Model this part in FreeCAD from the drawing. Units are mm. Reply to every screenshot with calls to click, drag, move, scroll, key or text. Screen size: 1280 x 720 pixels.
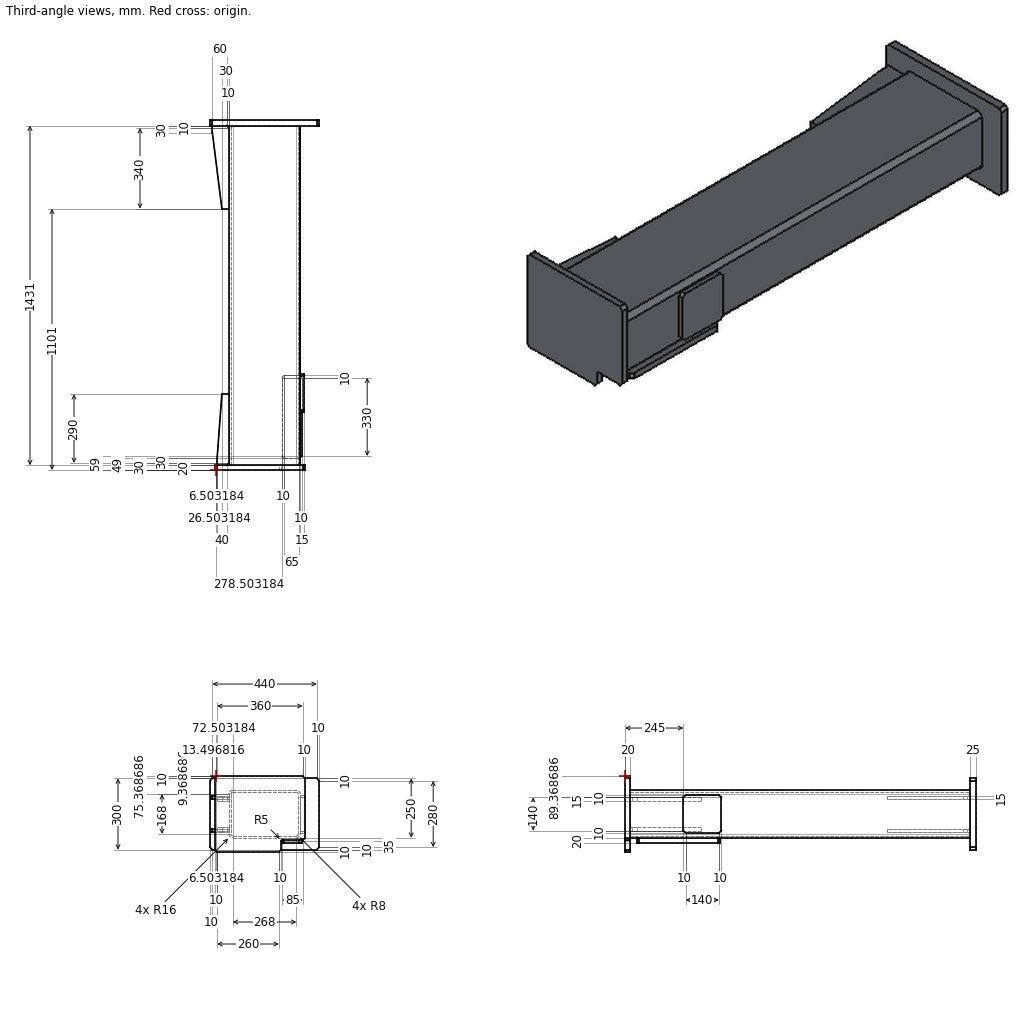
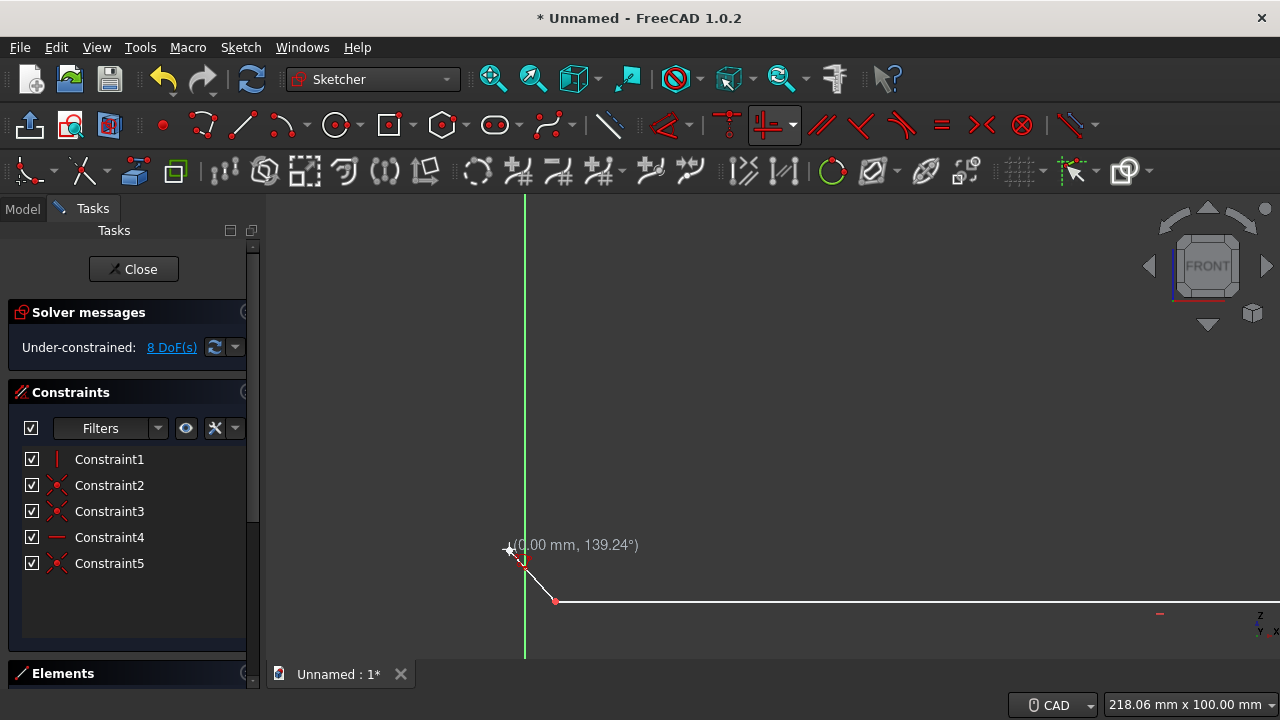
scroll(530, 572, down, 8)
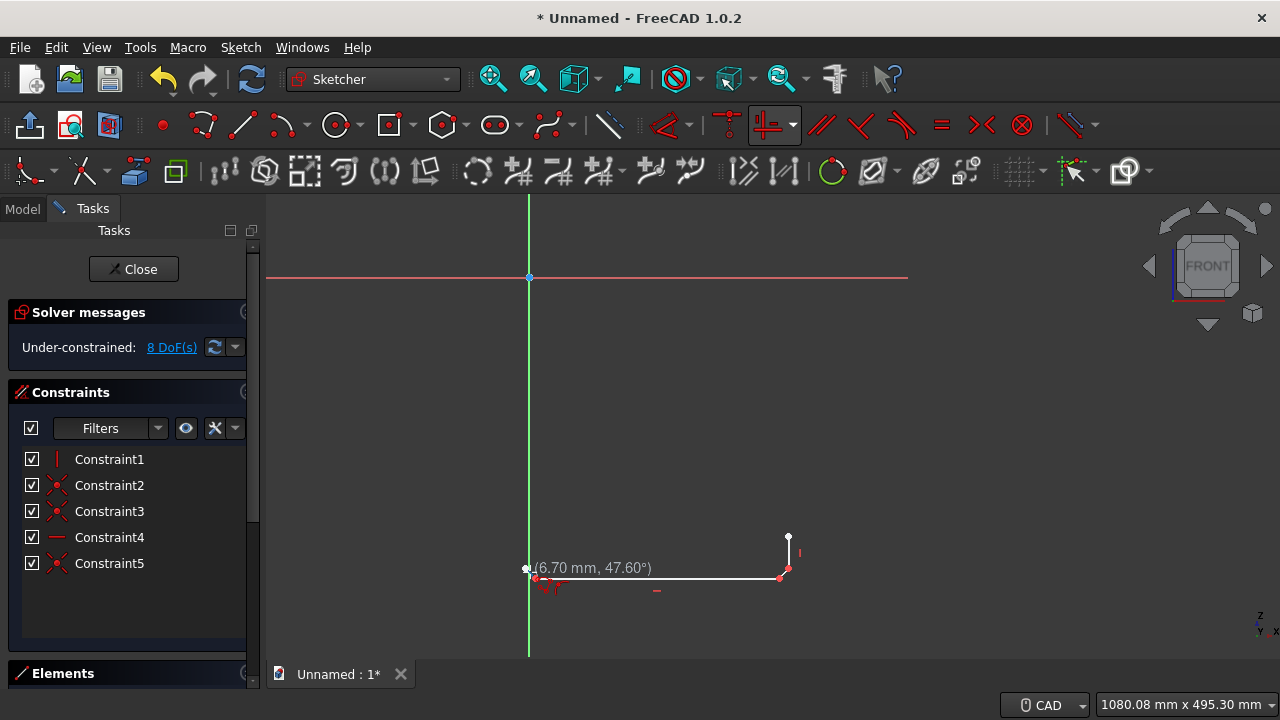
scroll(526, 286, up, 8)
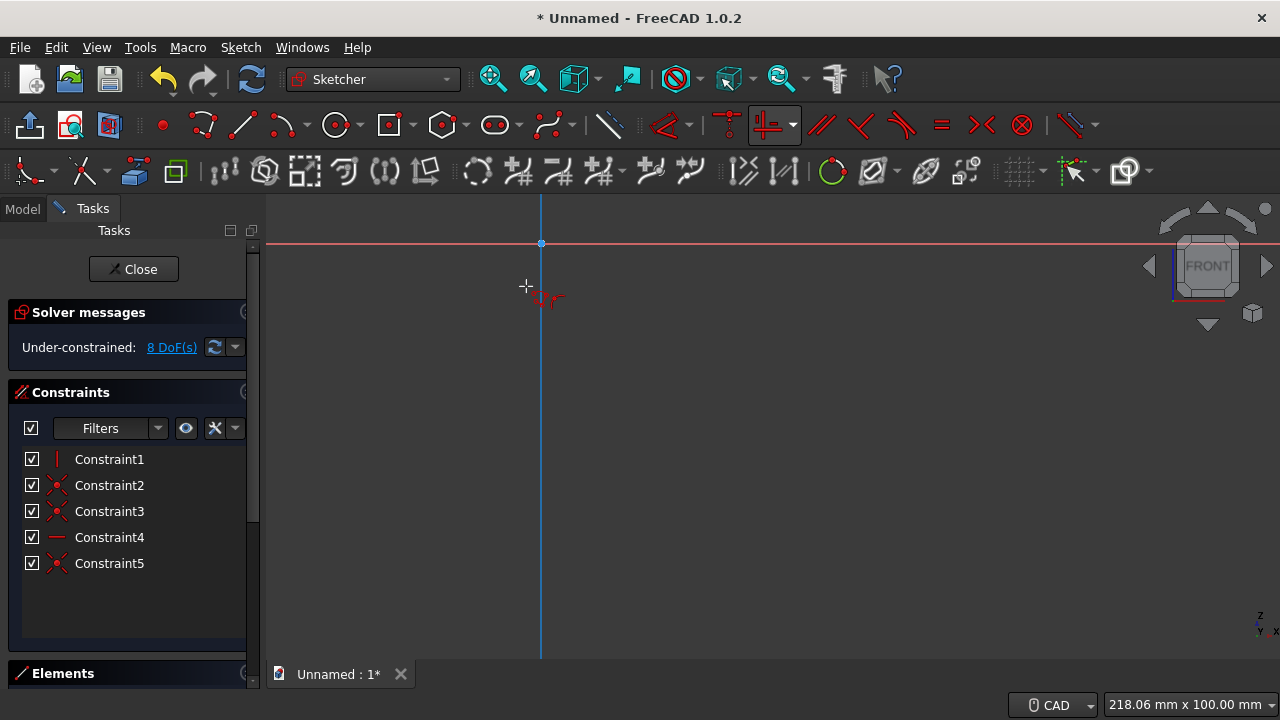
click(525, 287)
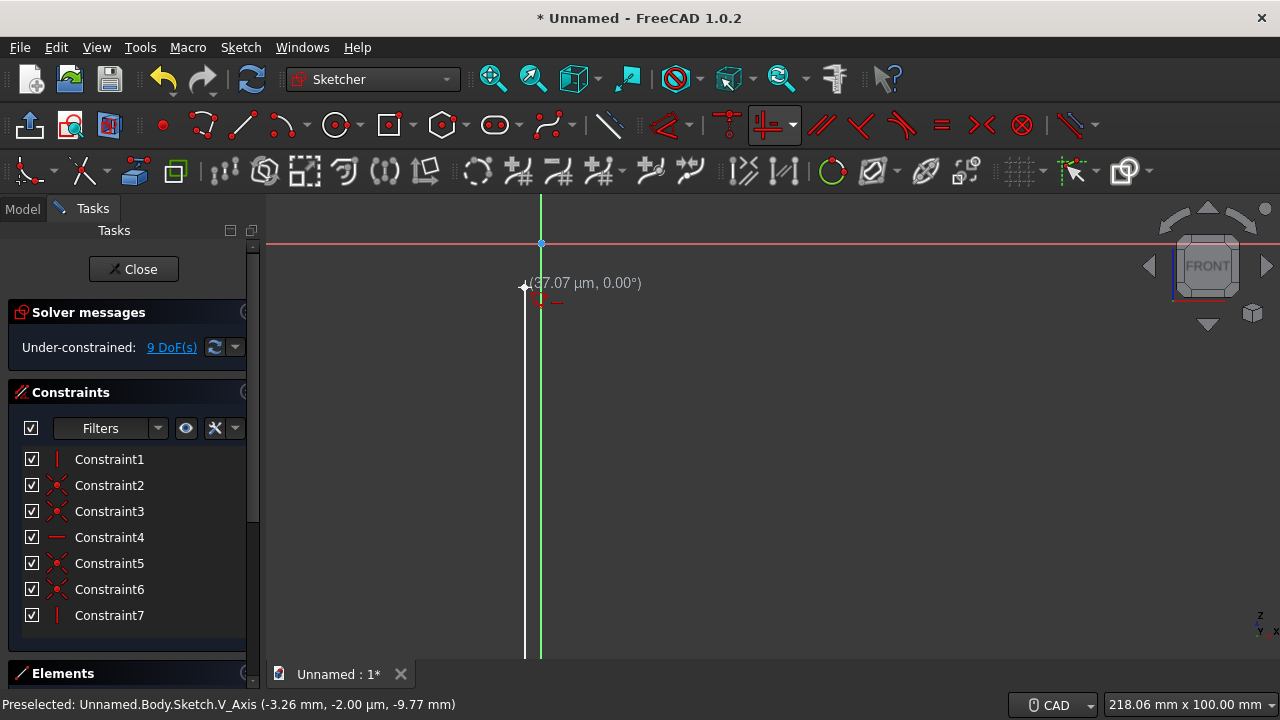
scroll(571, 241, up, 9)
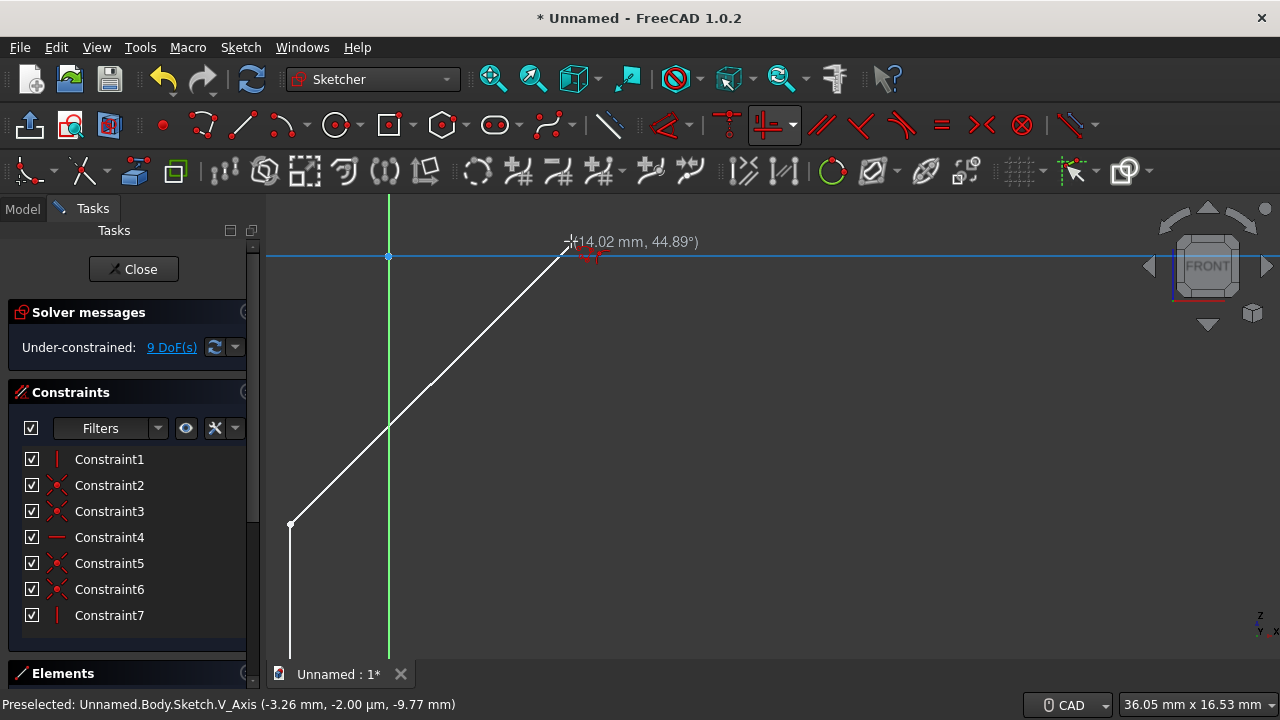
click(572, 238)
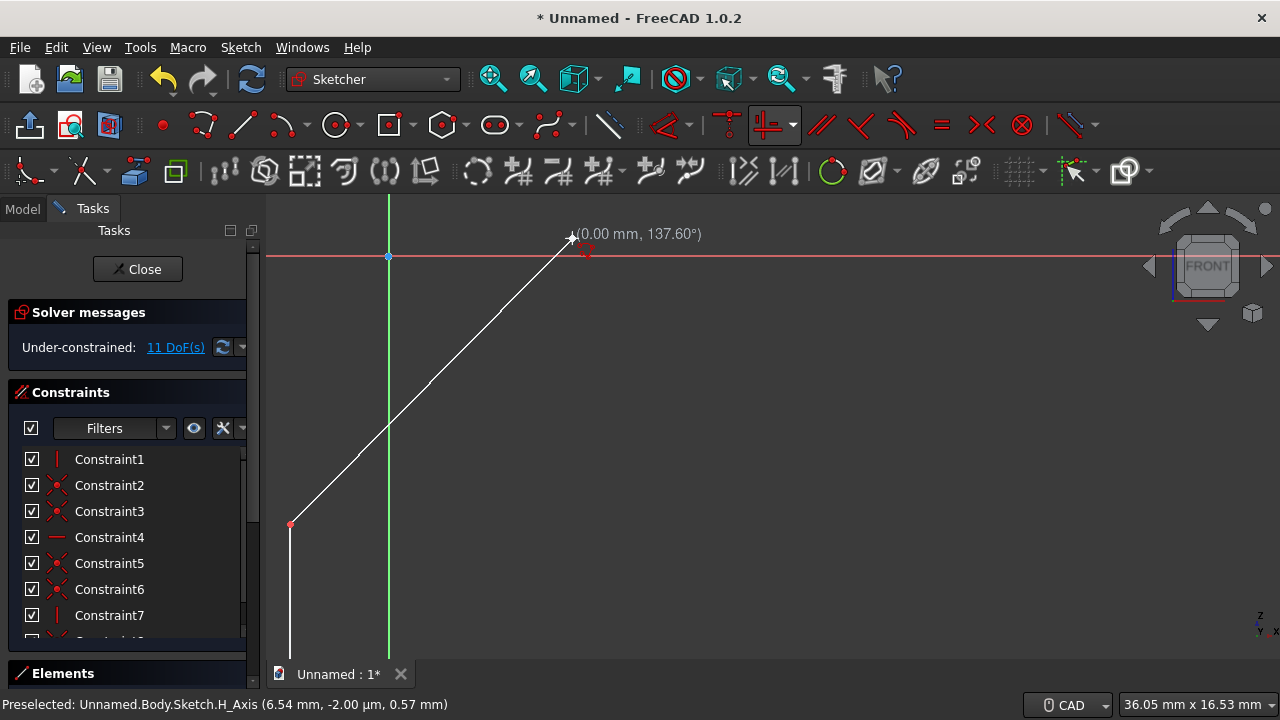
scroll(534, 278, down, 17)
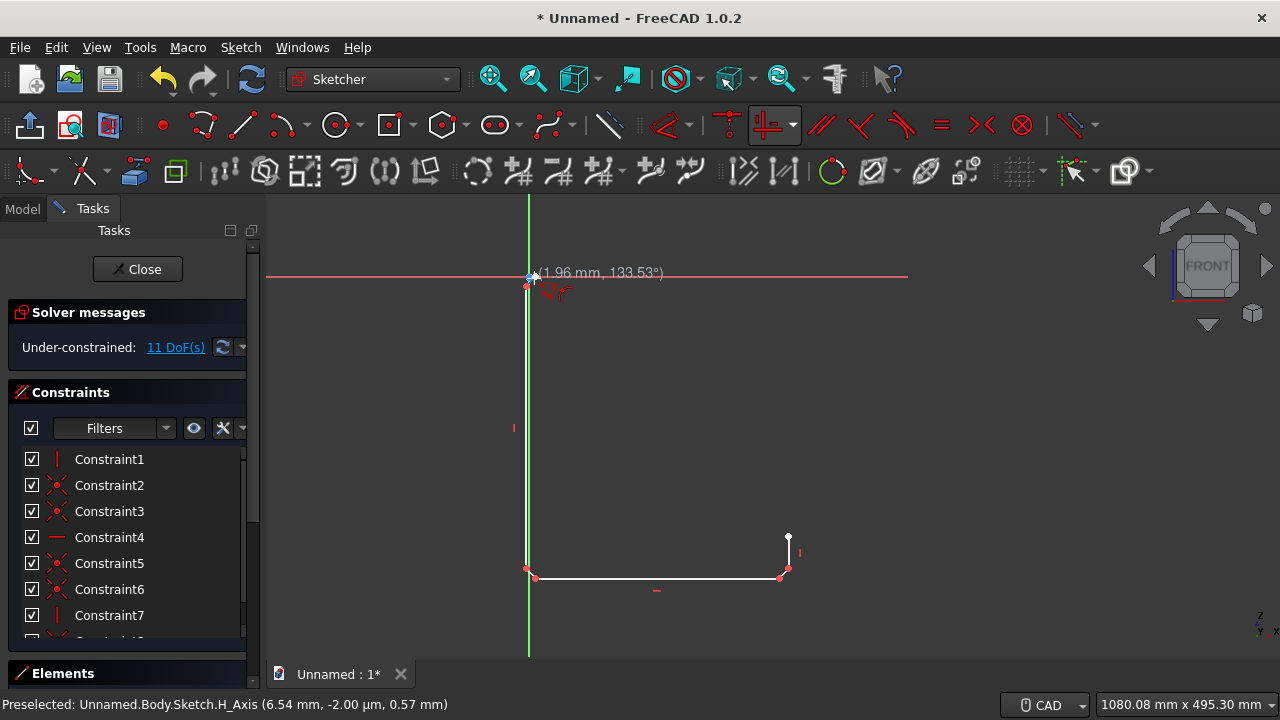
scroll(873, 277, up, 17)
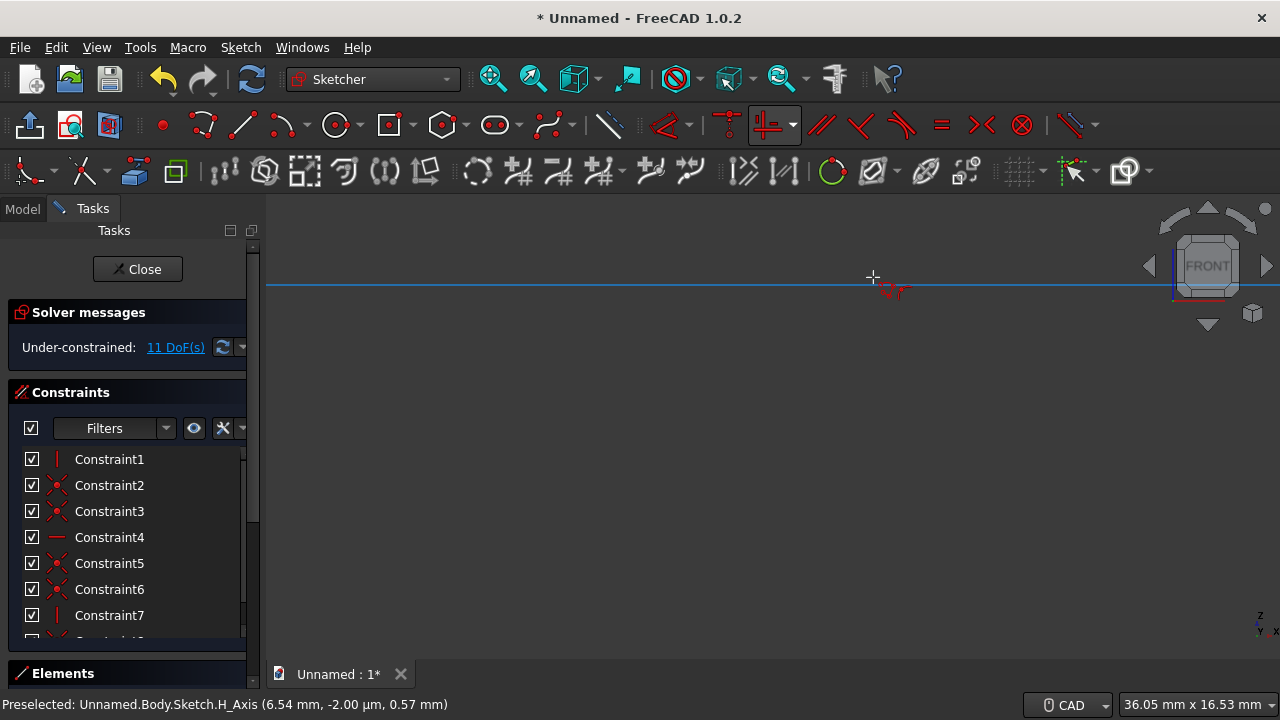
click(870, 267)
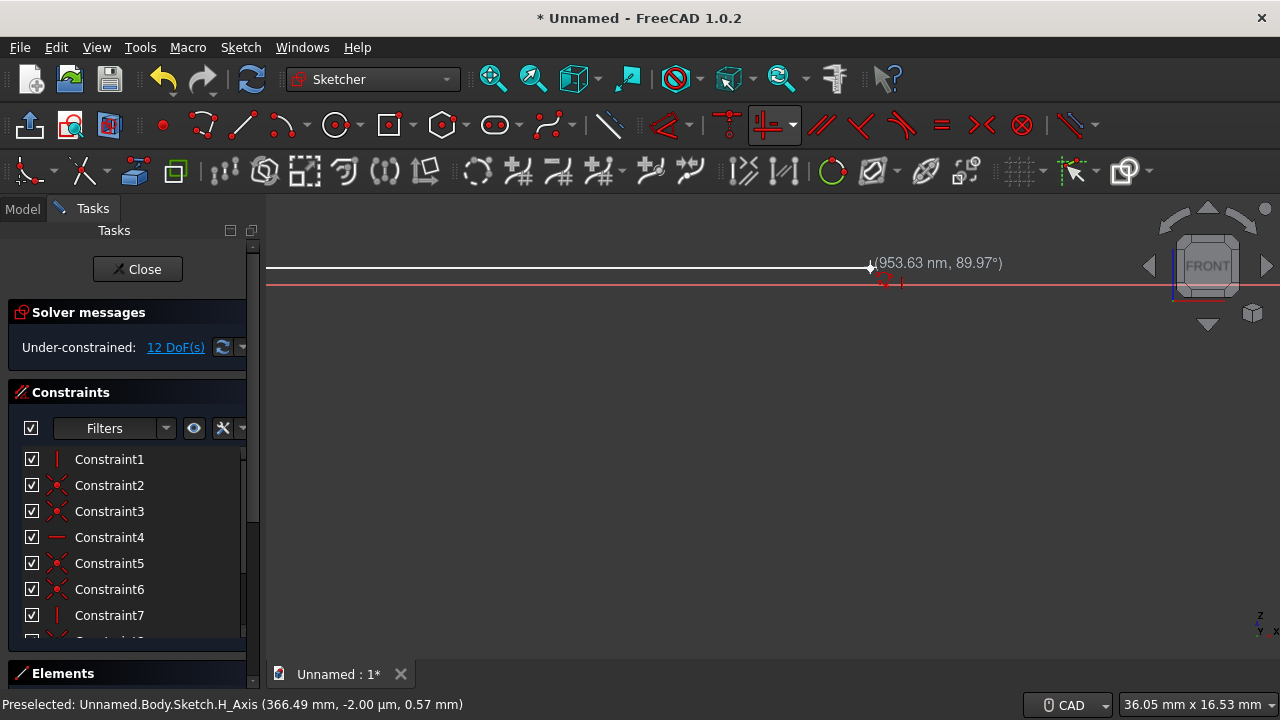
scroll(874, 277, down, 17)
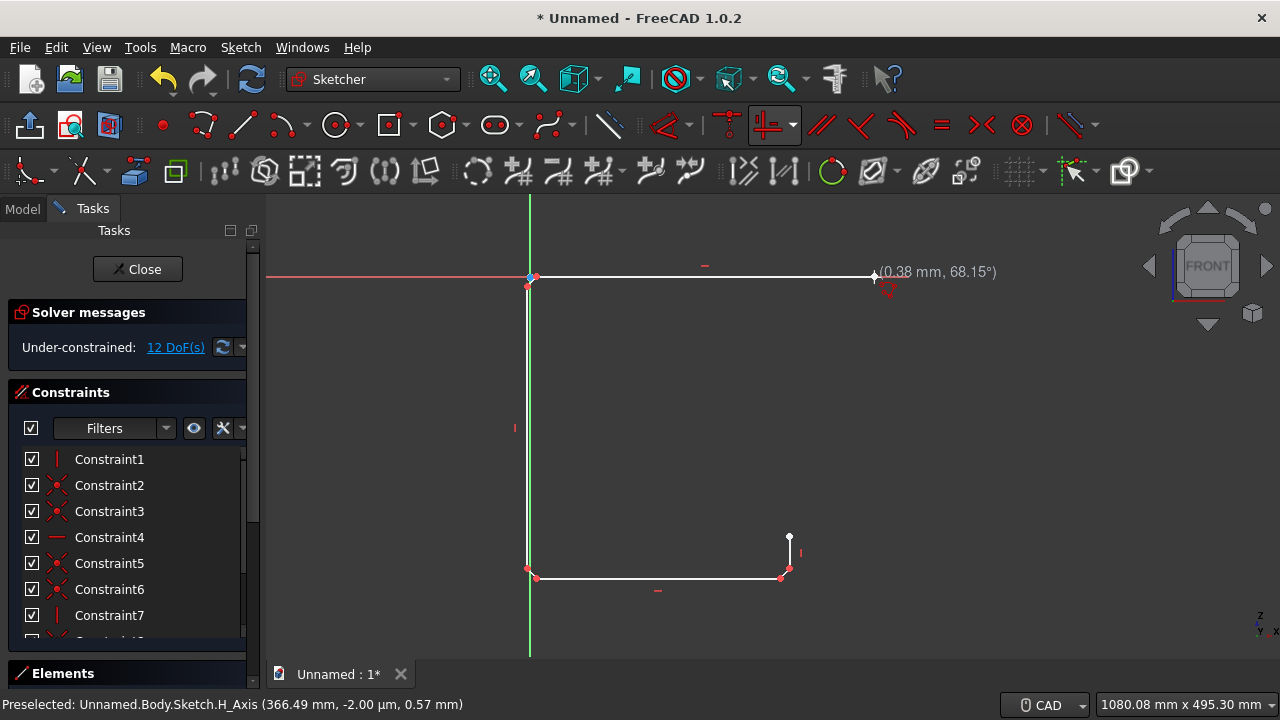
scroll(884, 286, up, 3)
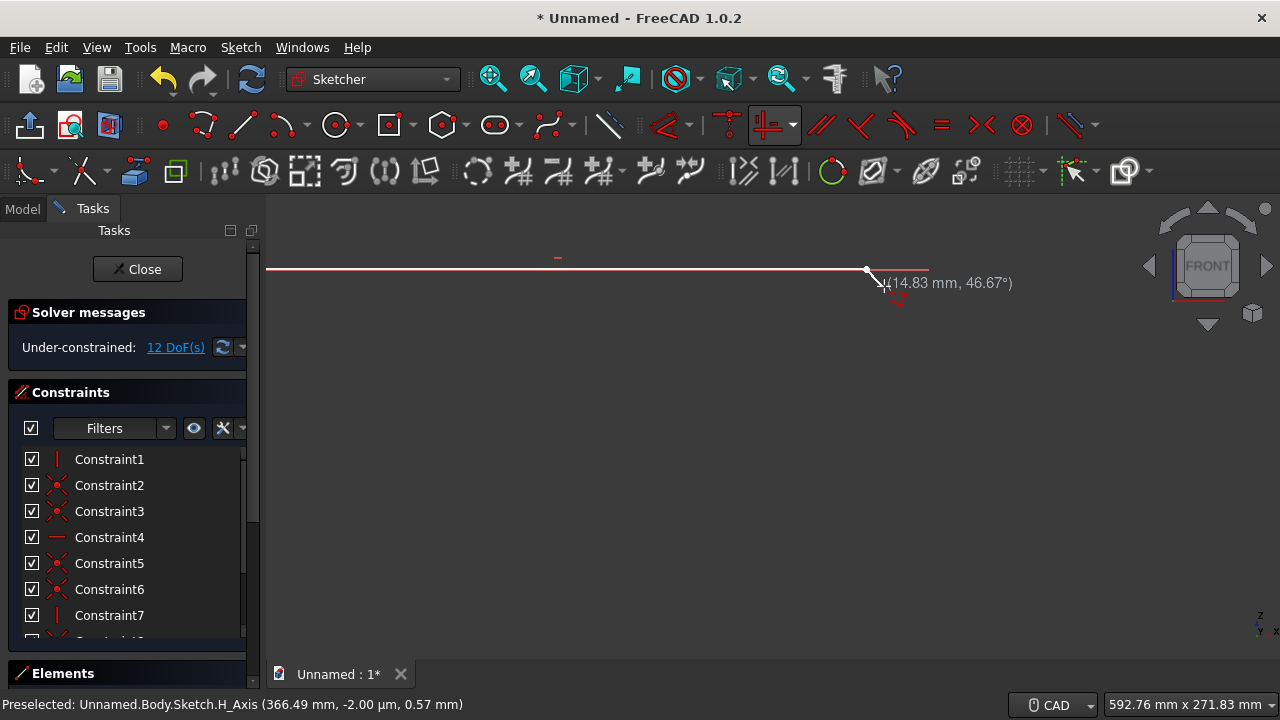
click(883, 286)